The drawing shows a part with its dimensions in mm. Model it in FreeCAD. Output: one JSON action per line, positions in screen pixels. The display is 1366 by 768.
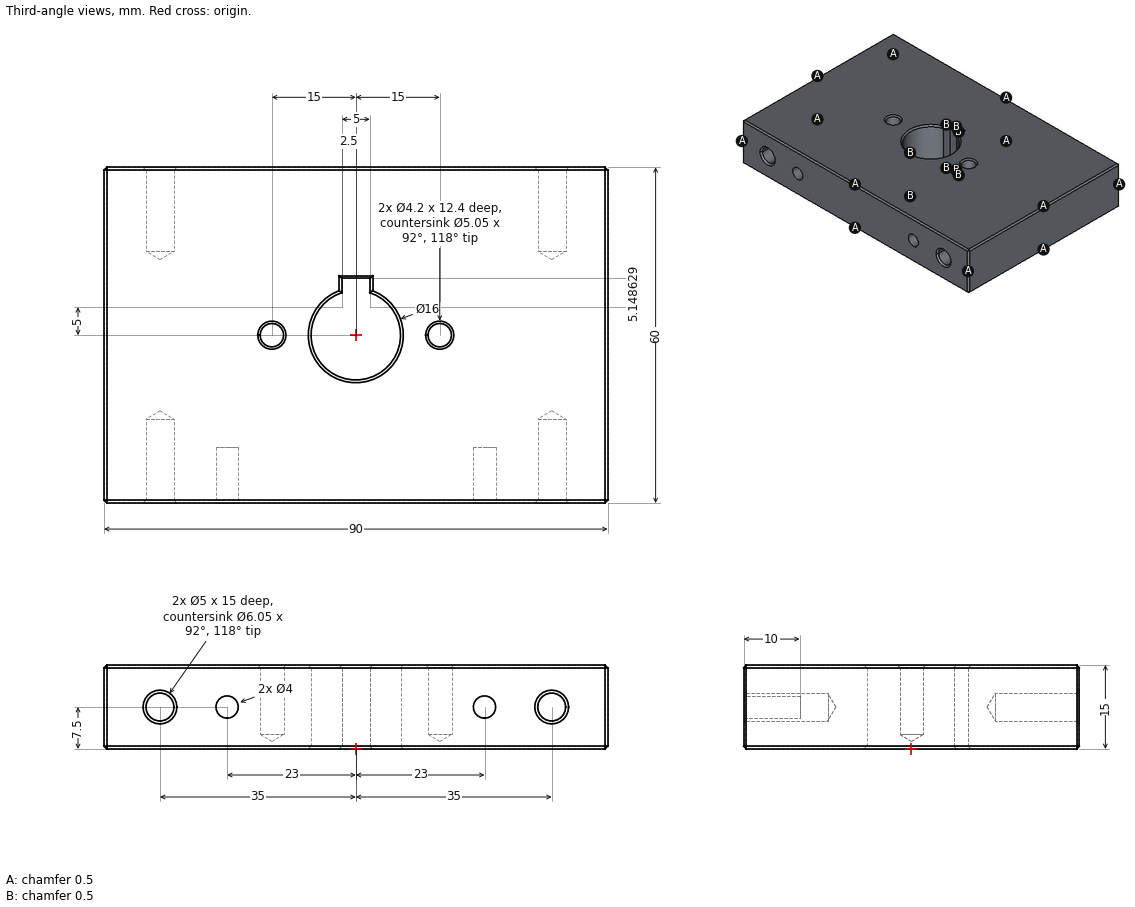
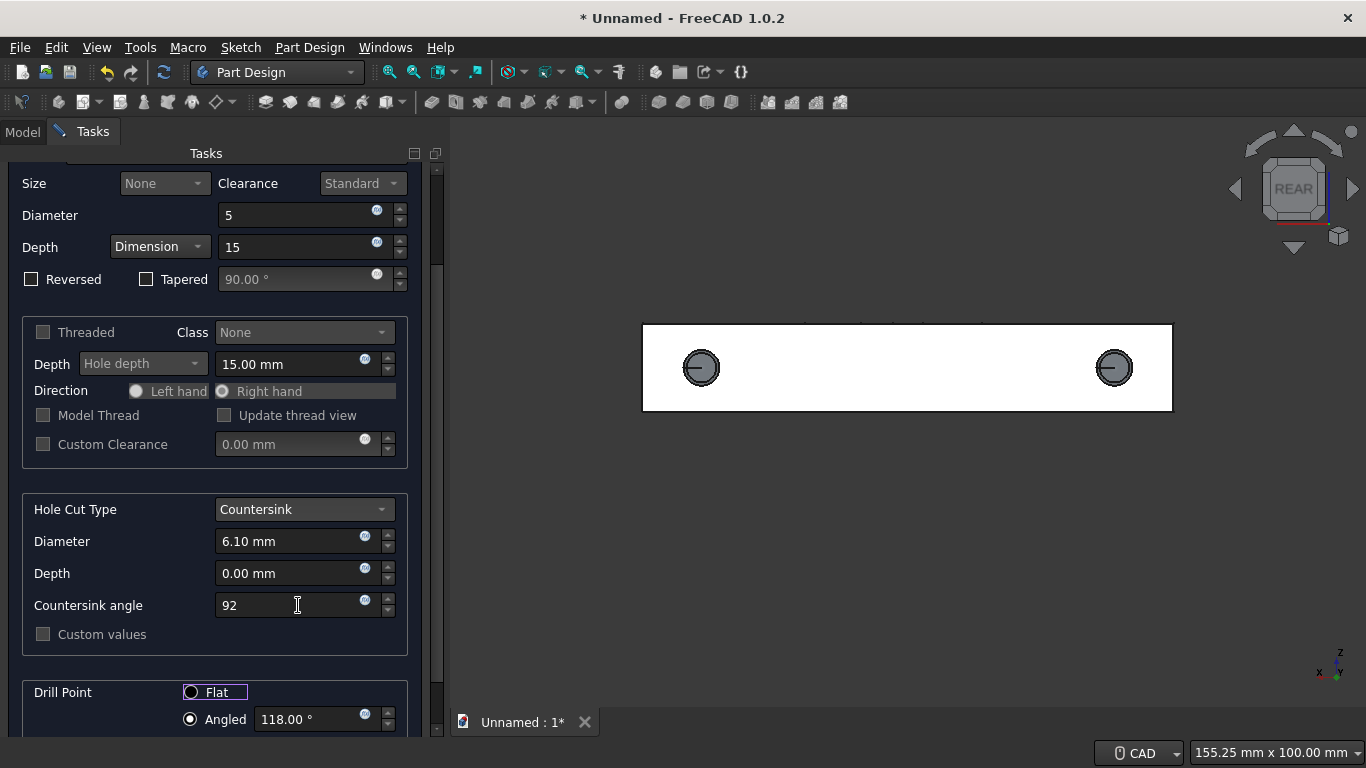
{"action": "triple_click", "coordinate": [298, 541]}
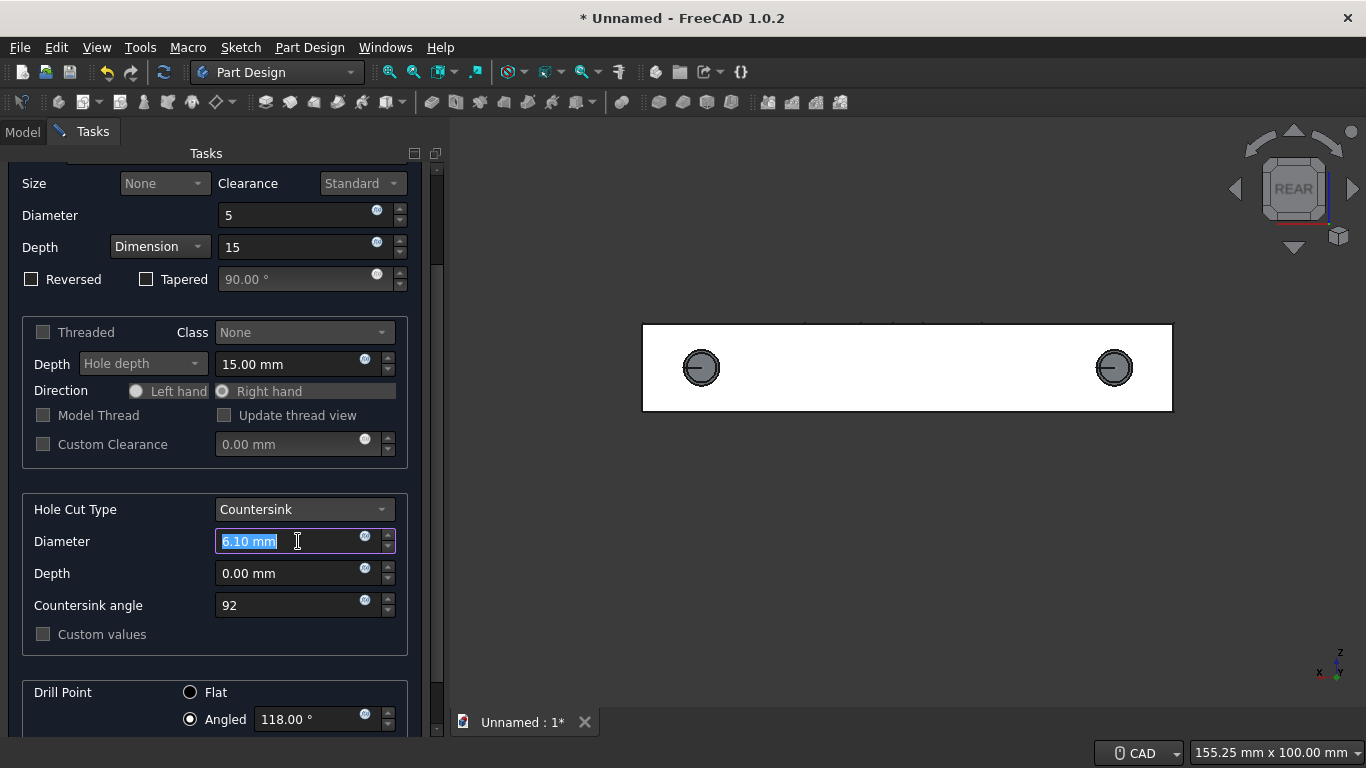
{"action": "type", "text": "6.05"}
{"action": "key", "text": "Tab"}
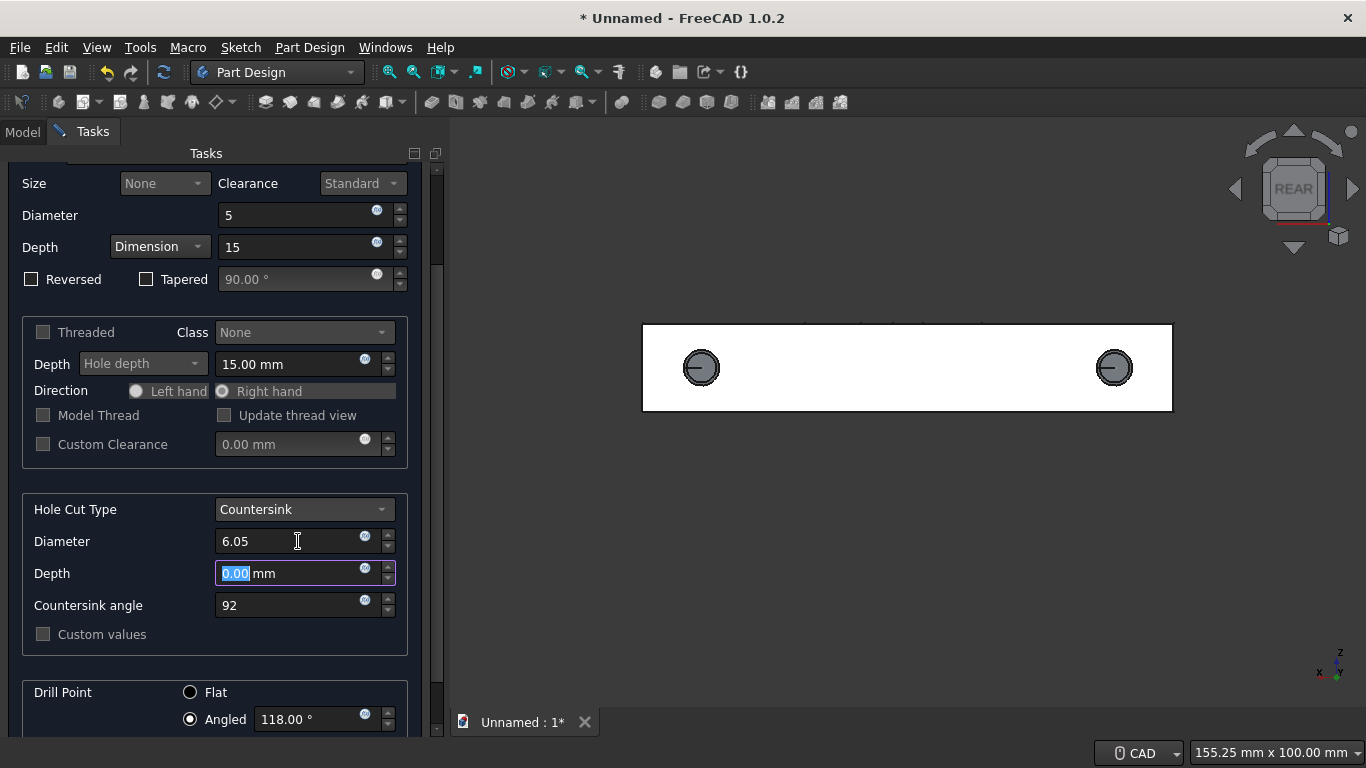
{"action": "scroll", "coordinate": [437, 450], "scroll_direction": "up", "scroll_amount": 3}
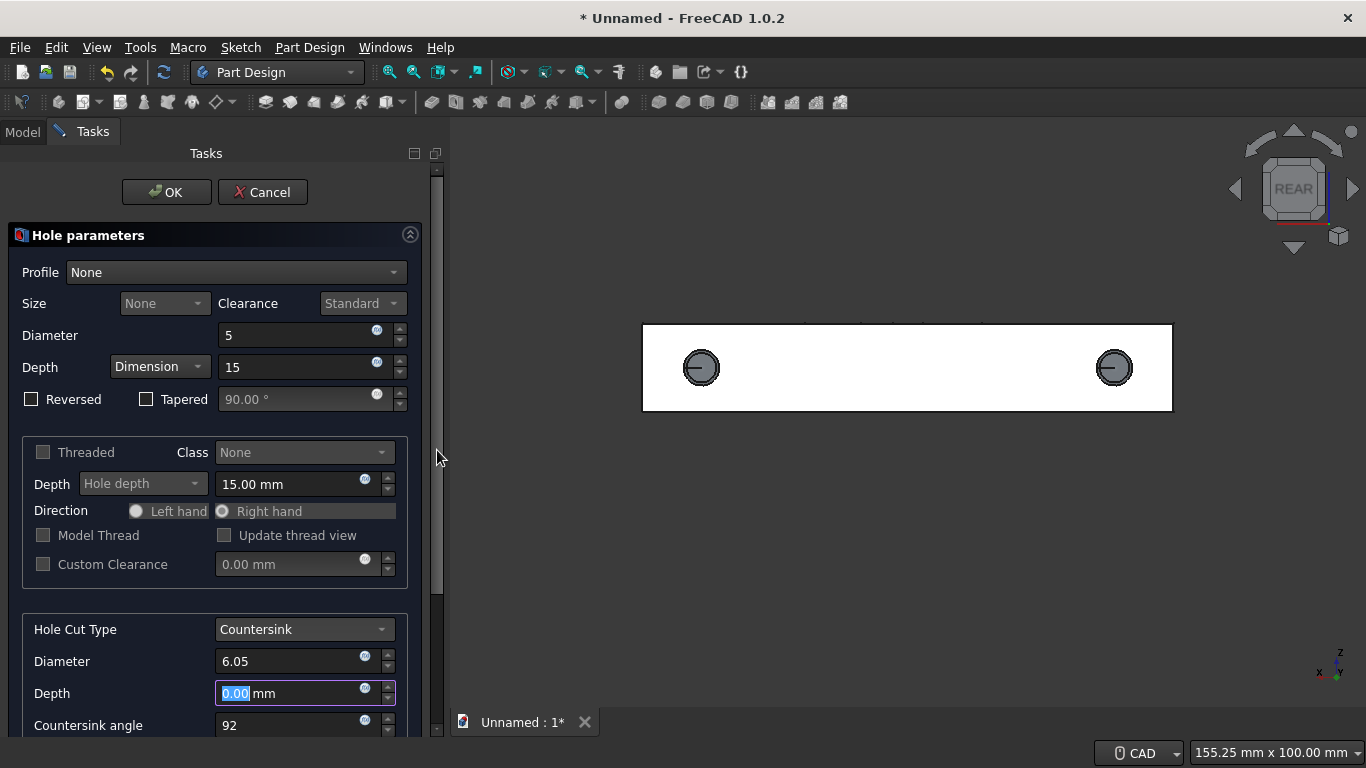
{"action": "left_click", "coordinate": [167, 192]}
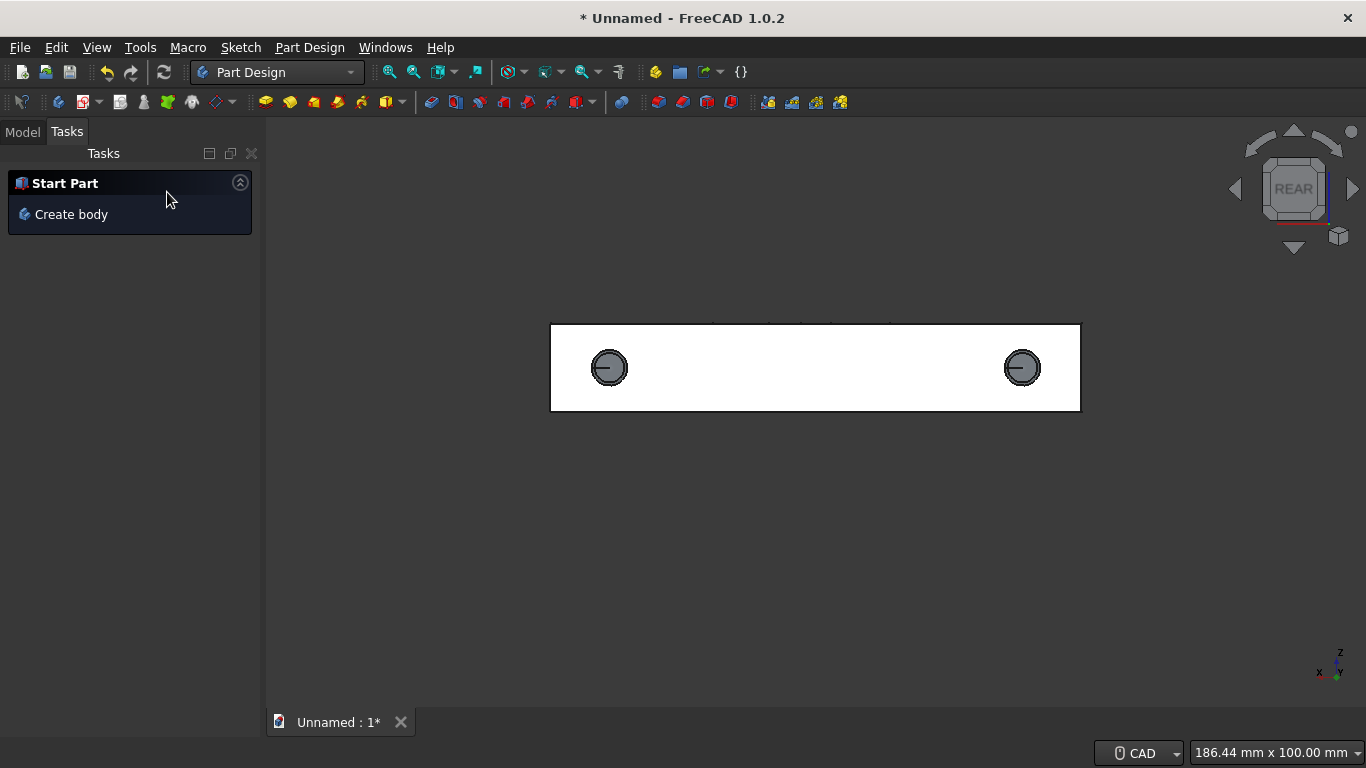
{"action": "key", "text": "0"}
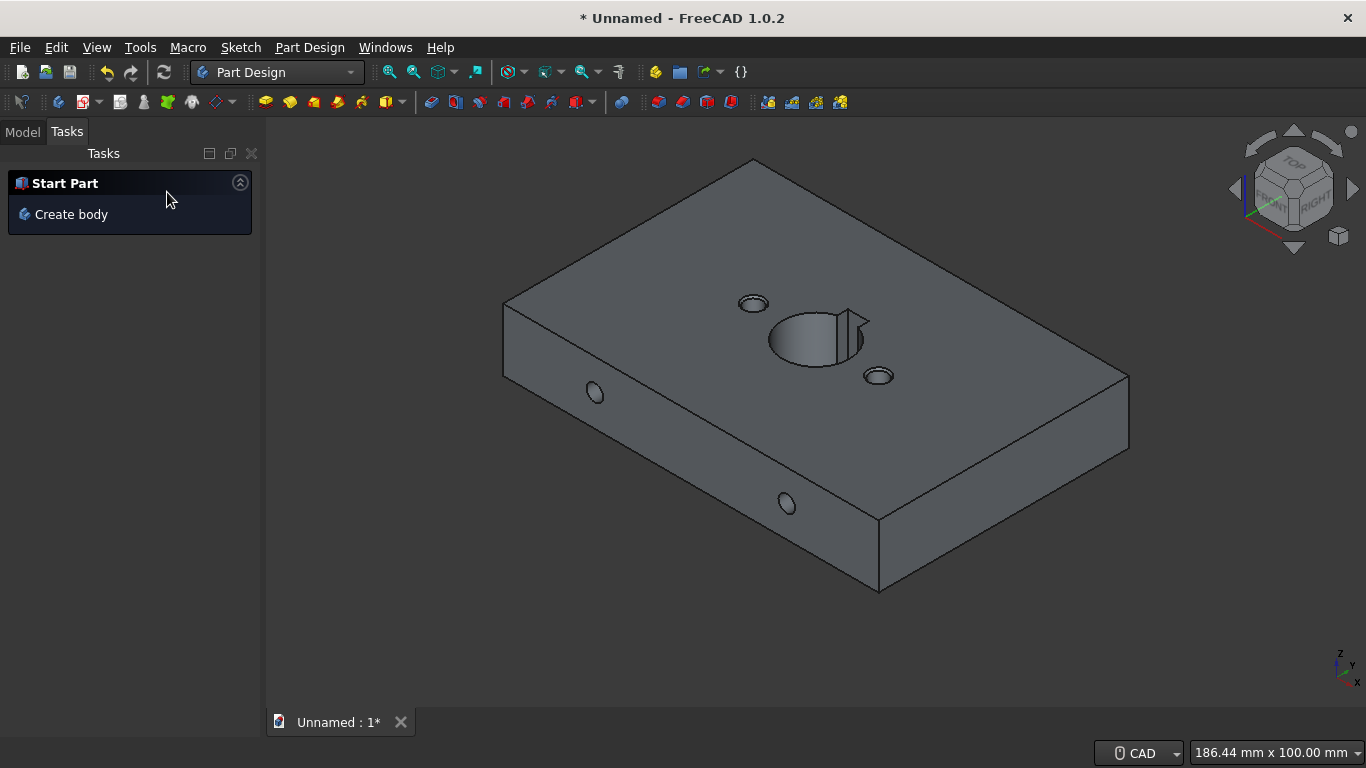
{"action": "left_click", "coordinate": [744, 478]}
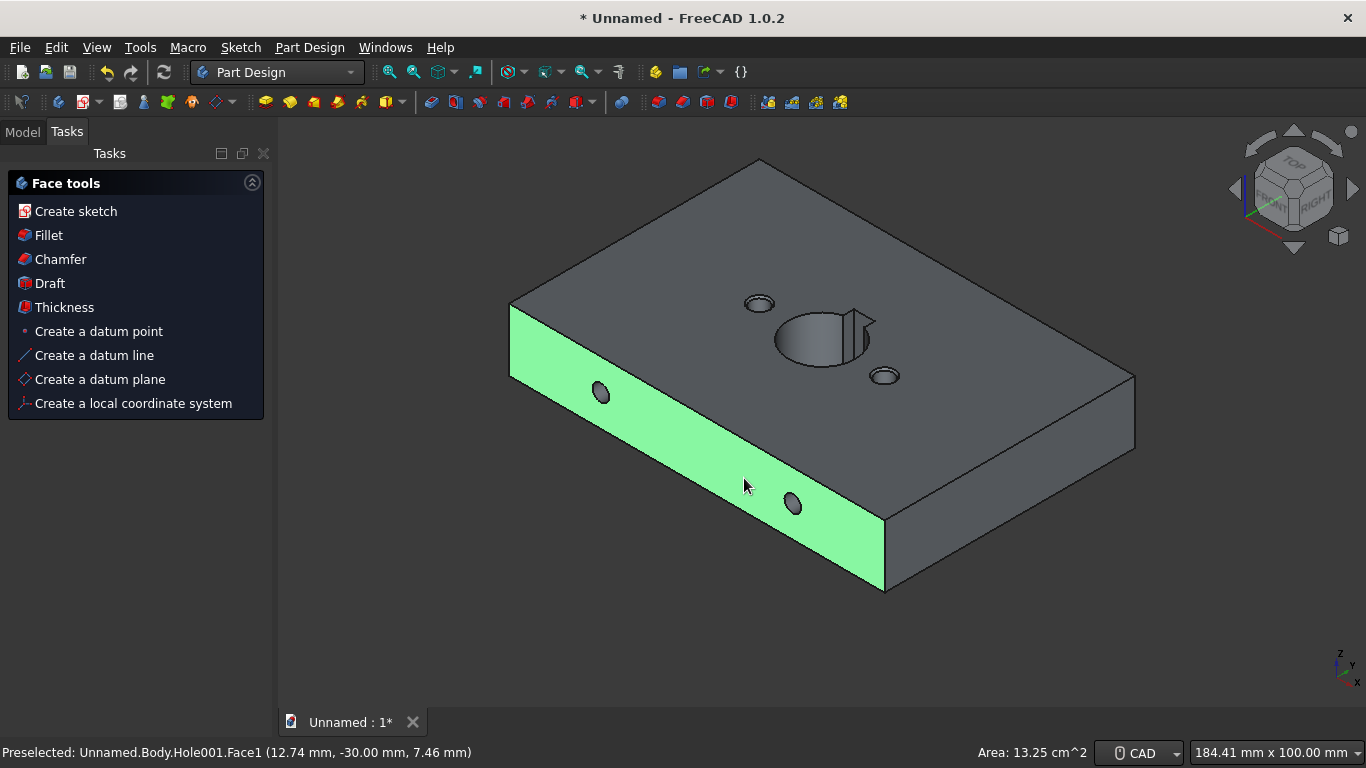
{"action": "left_click", "coordinate": [84, 102]}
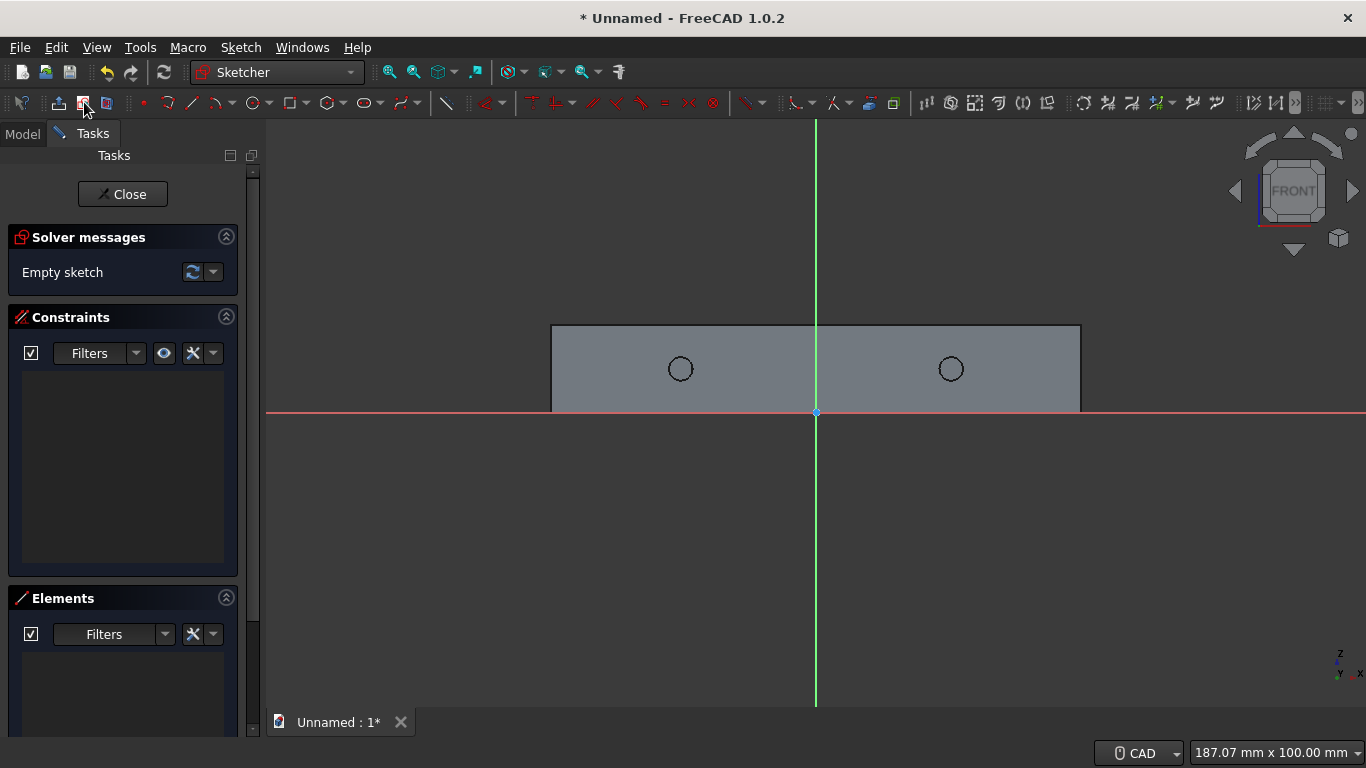
{"action": "scroll", "coordinate": [955, 324], "scroll_direction": "up", "scroll_amount": 2}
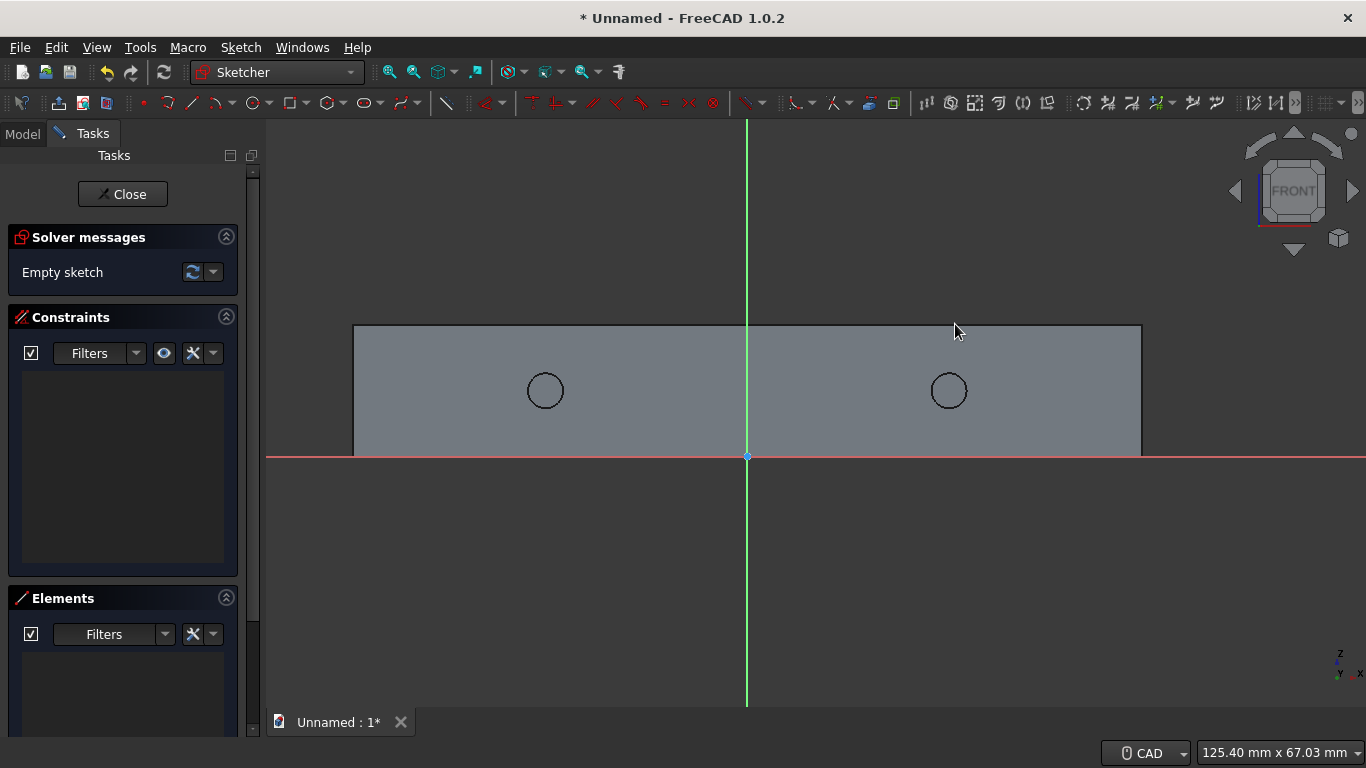
{"action": "key", "text": "g c"}